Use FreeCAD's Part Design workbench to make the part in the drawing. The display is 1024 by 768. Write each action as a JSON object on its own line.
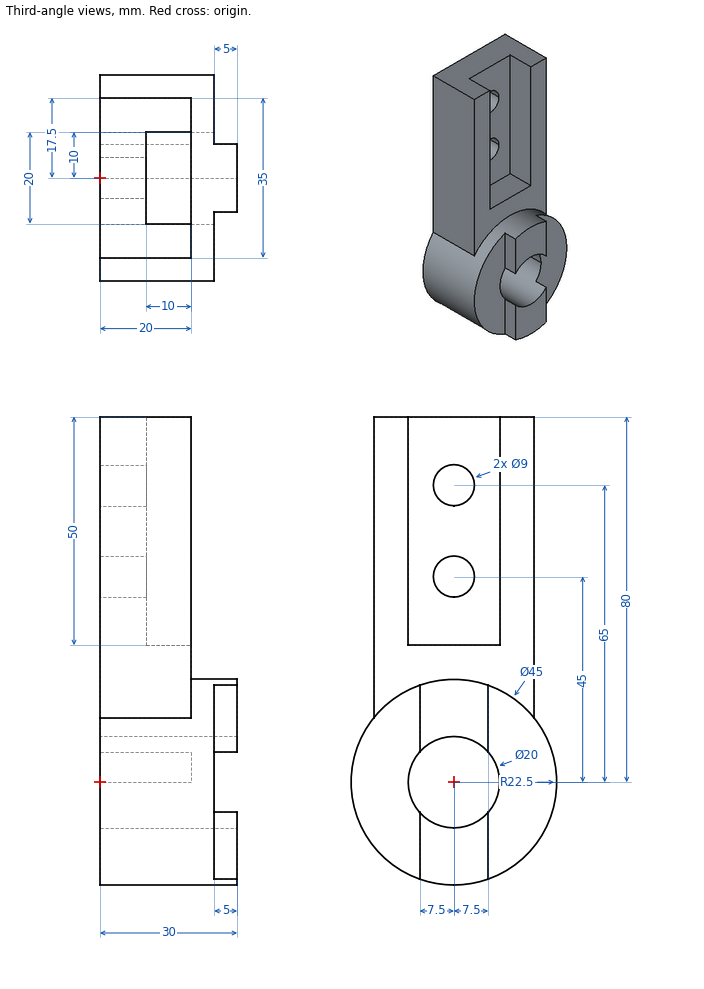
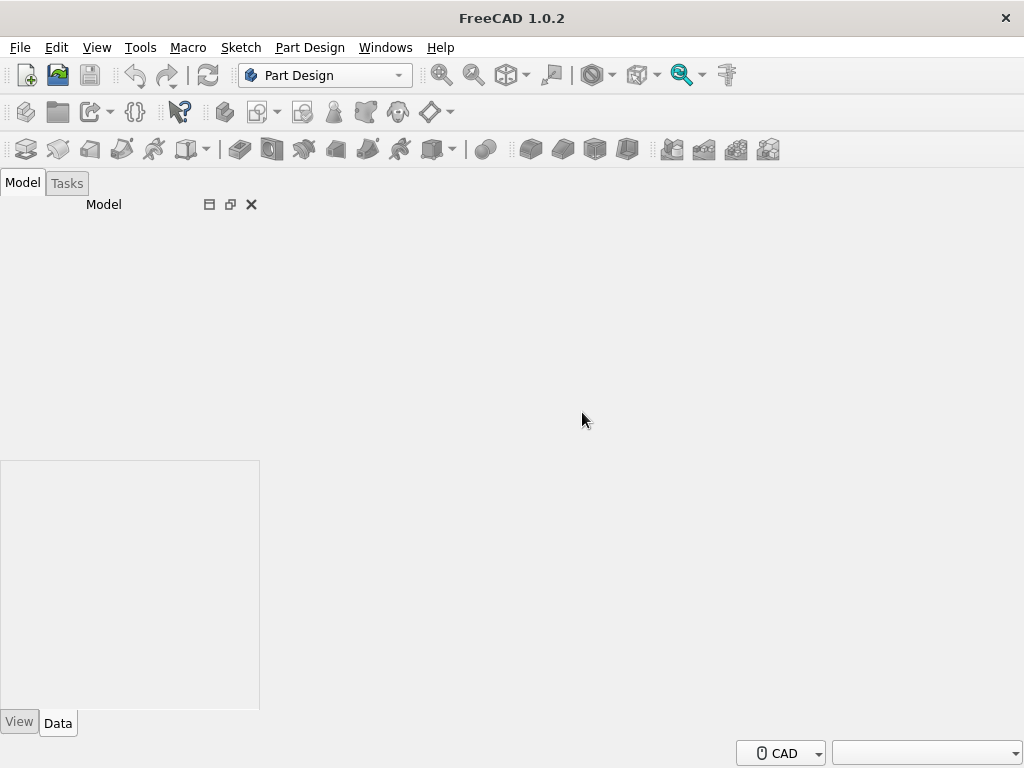
{"action": "left_click", "coordinate": [26, 76]}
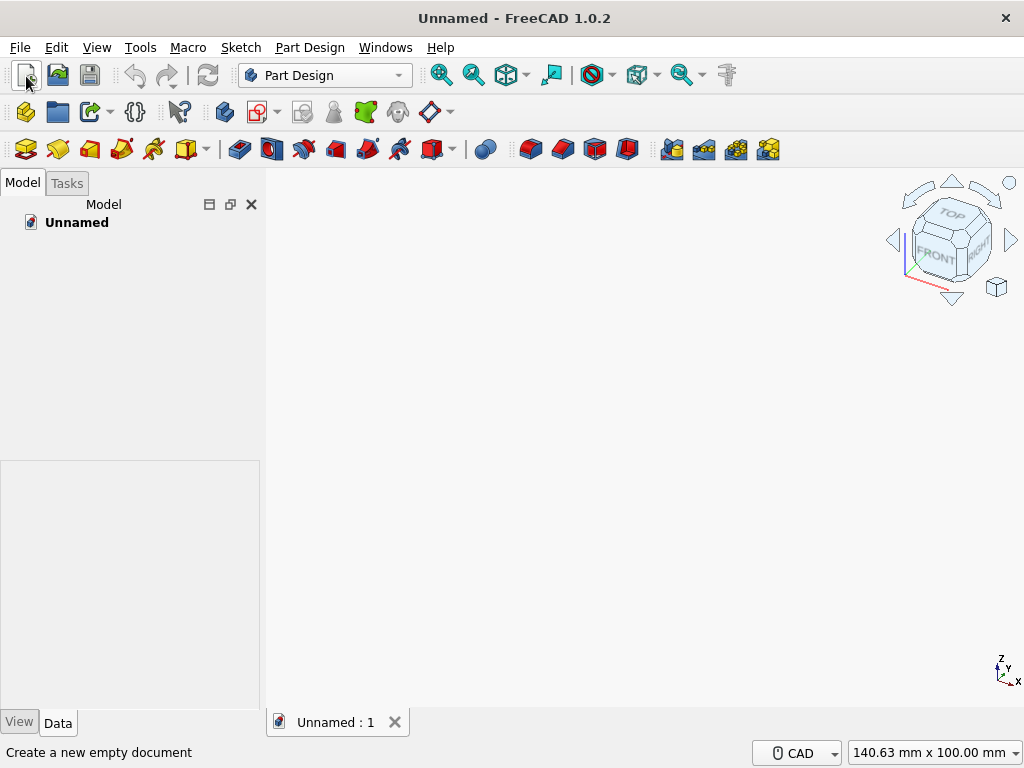
{"action": "left_click", "coordinate": [258, 112]}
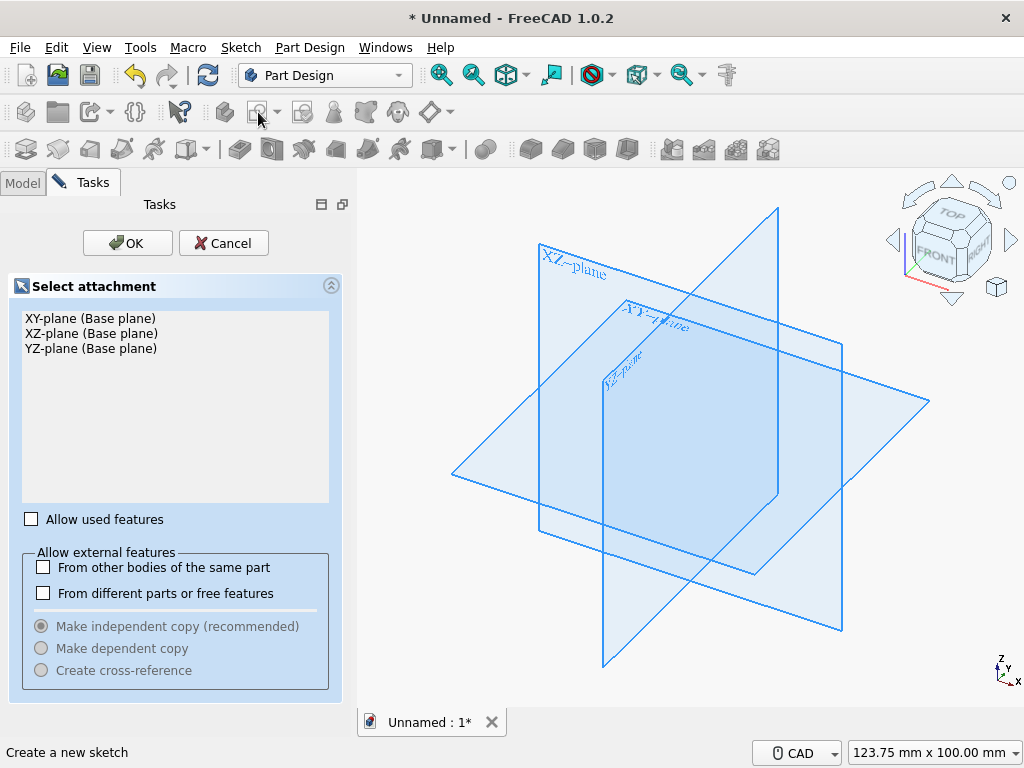
{"action": "left_click", "coordinate": [82, 348]}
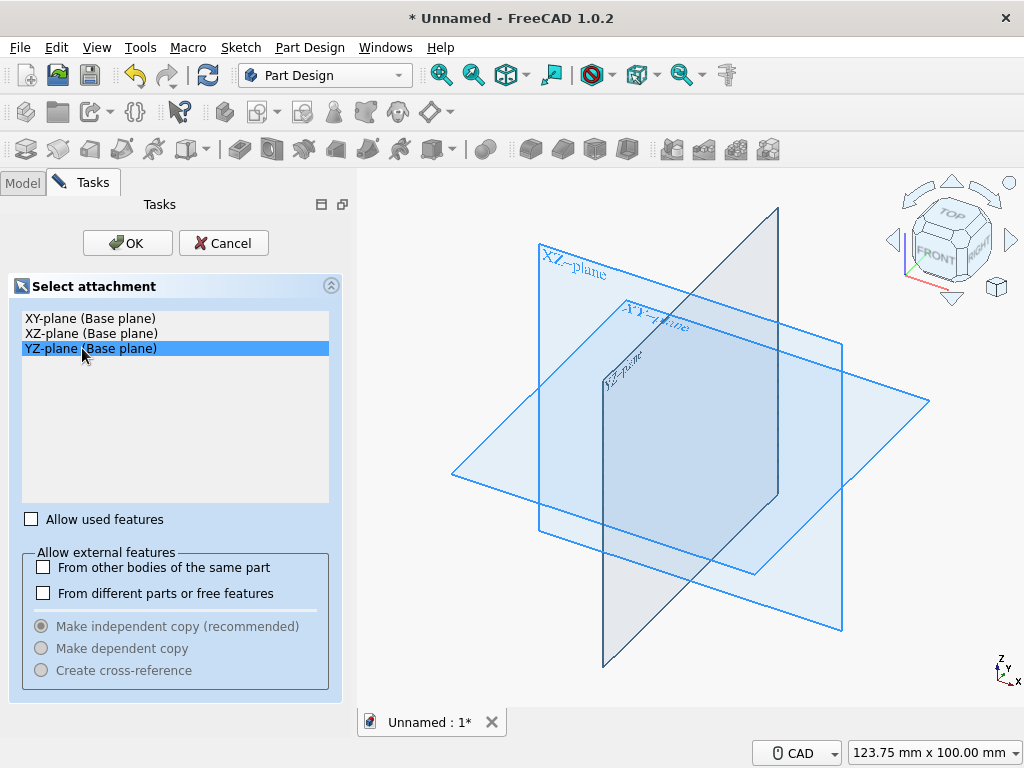
{"action": "left_click", "coordinate": [128, 243]}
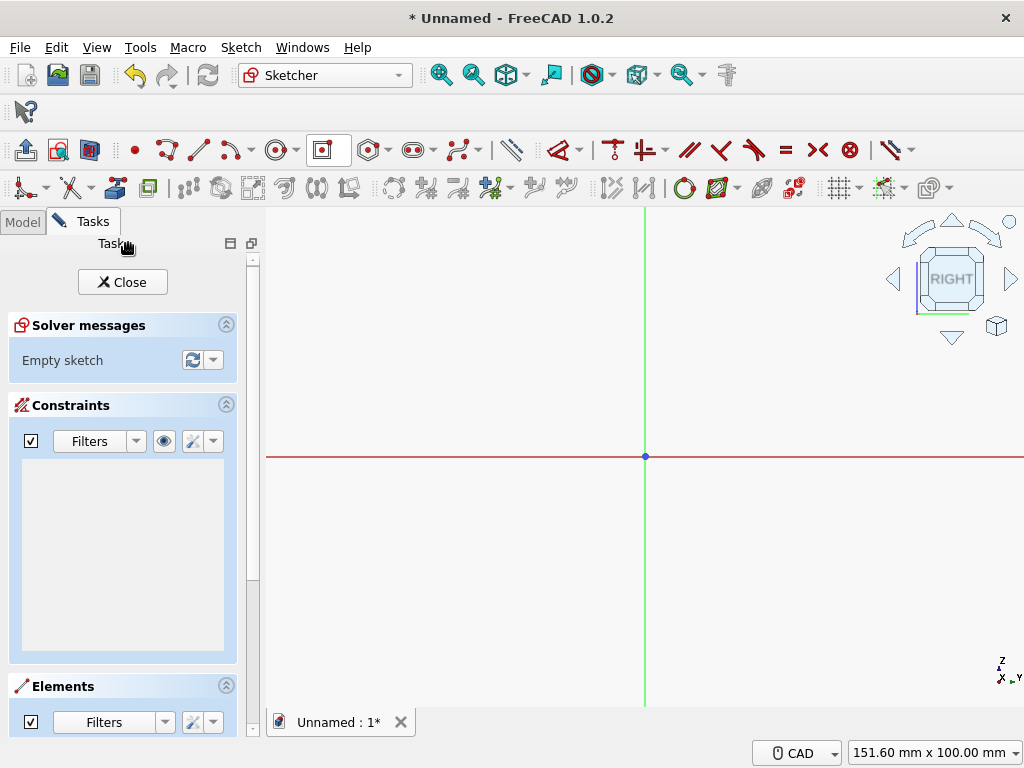
{"action": "scroll", "coordinate": [784, 457], "scroll_direction": "up", "scroll_amount": 2}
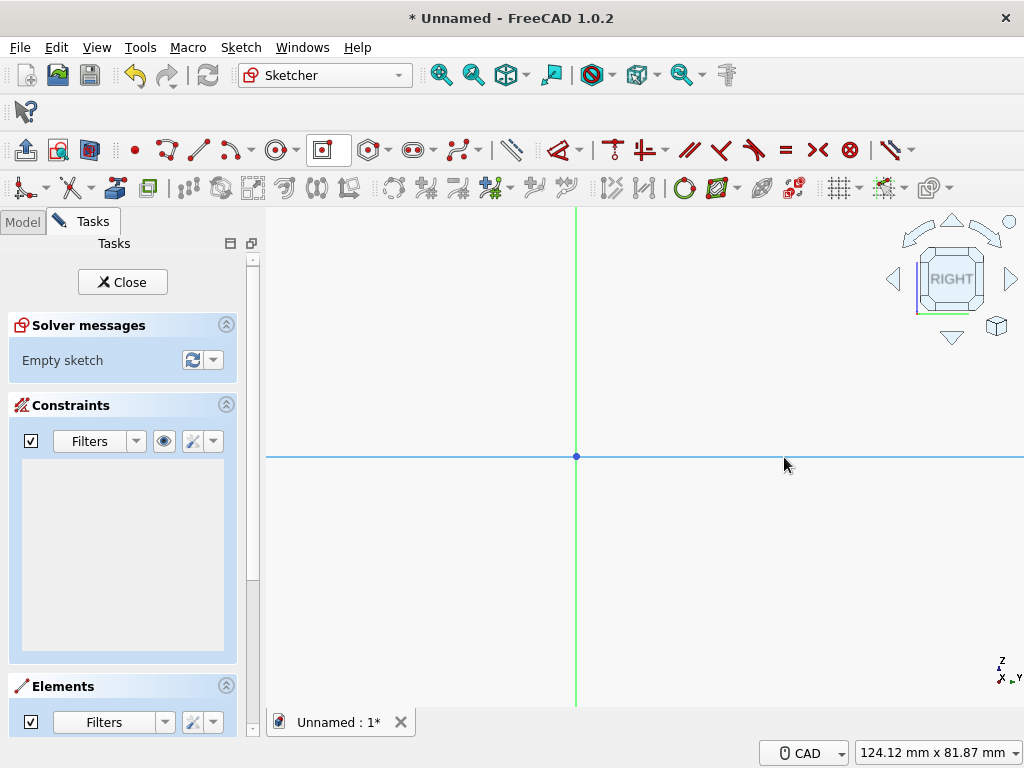
{"action": "left_click", "coordinate": [276, 150]}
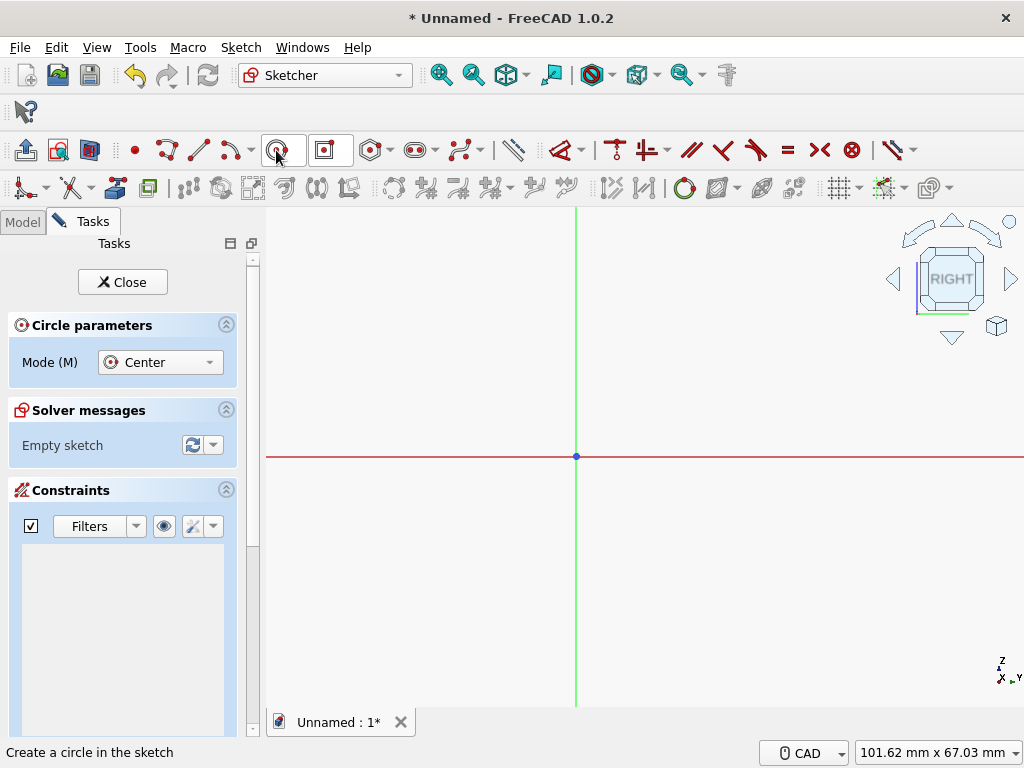
{"action": "left_click", "coordinate": [576, 457]}
{"action": "mouse_move", "coordinate": [695, 338]}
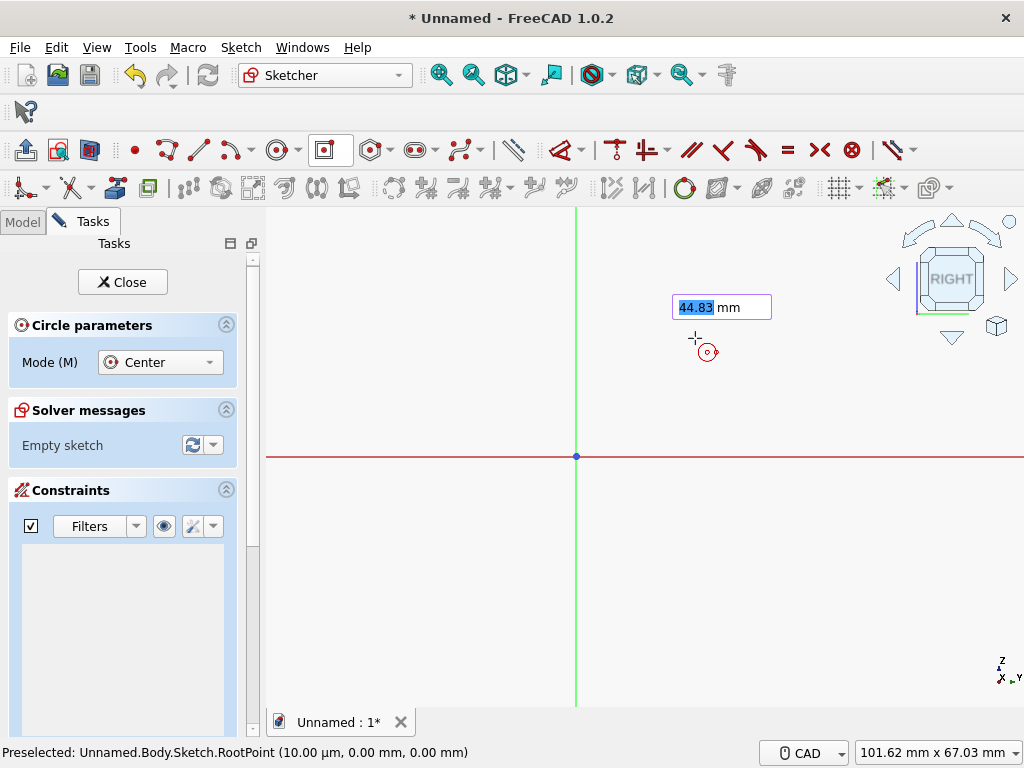
{"action": "type", "text": "45"}
{"action": "key", "text": "Return"}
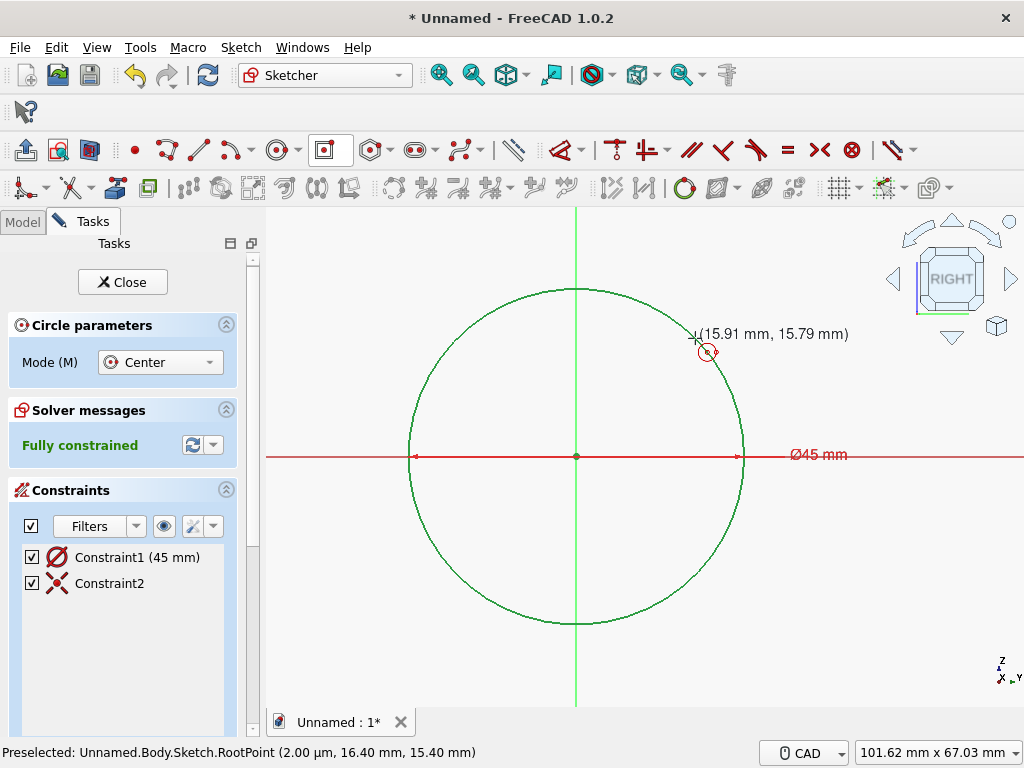
{"action": "left_click", "coordinate": [576, 457]}
{"action": "mouse_move", "coordinate": [629, 404]}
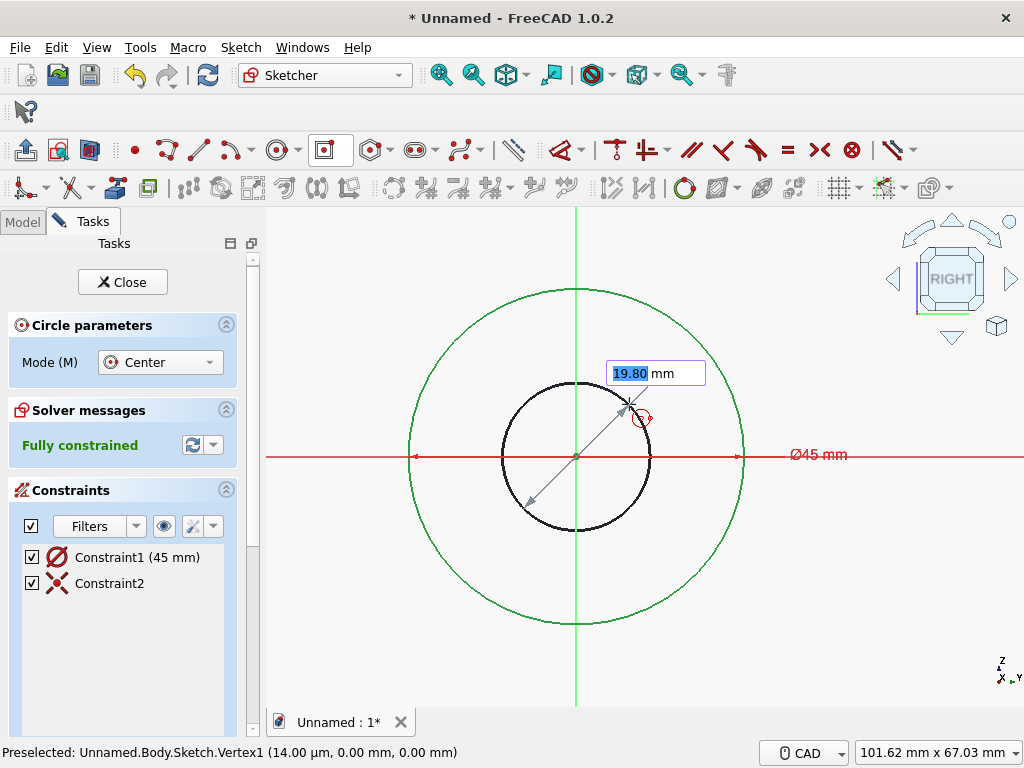
{"action": "type", "text": "20"}
{"action": "key", "text": "Return"}
{"action": "key", "text": "Escape"}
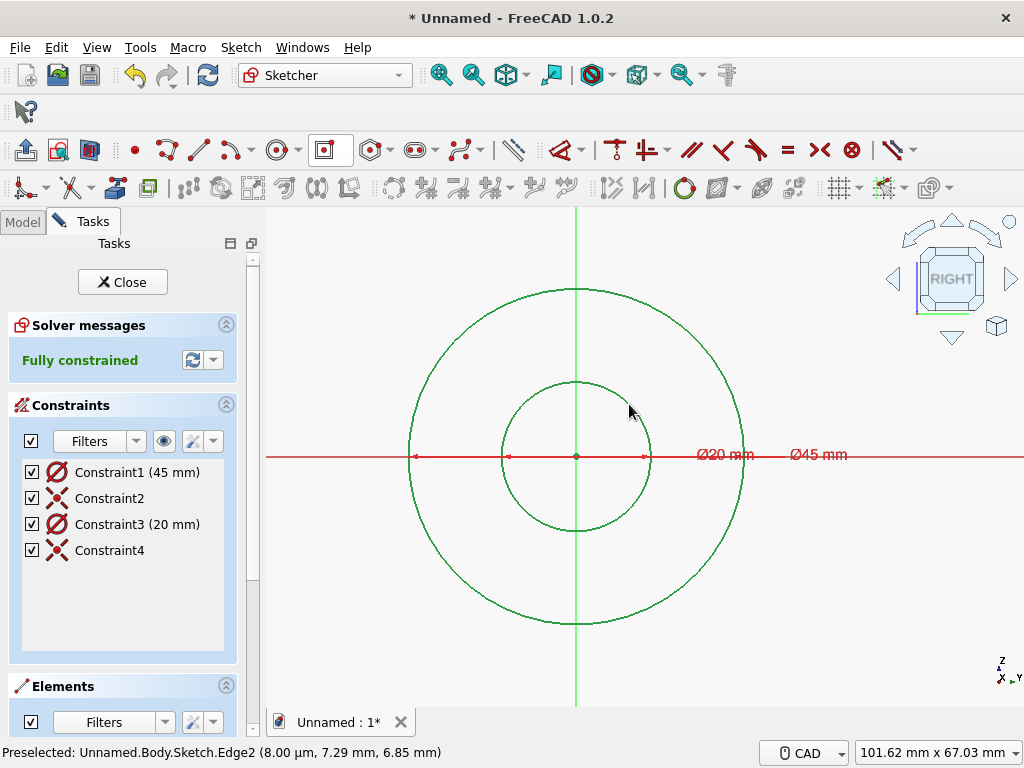
{"action": "left_click", "coordinate": [123, 282]}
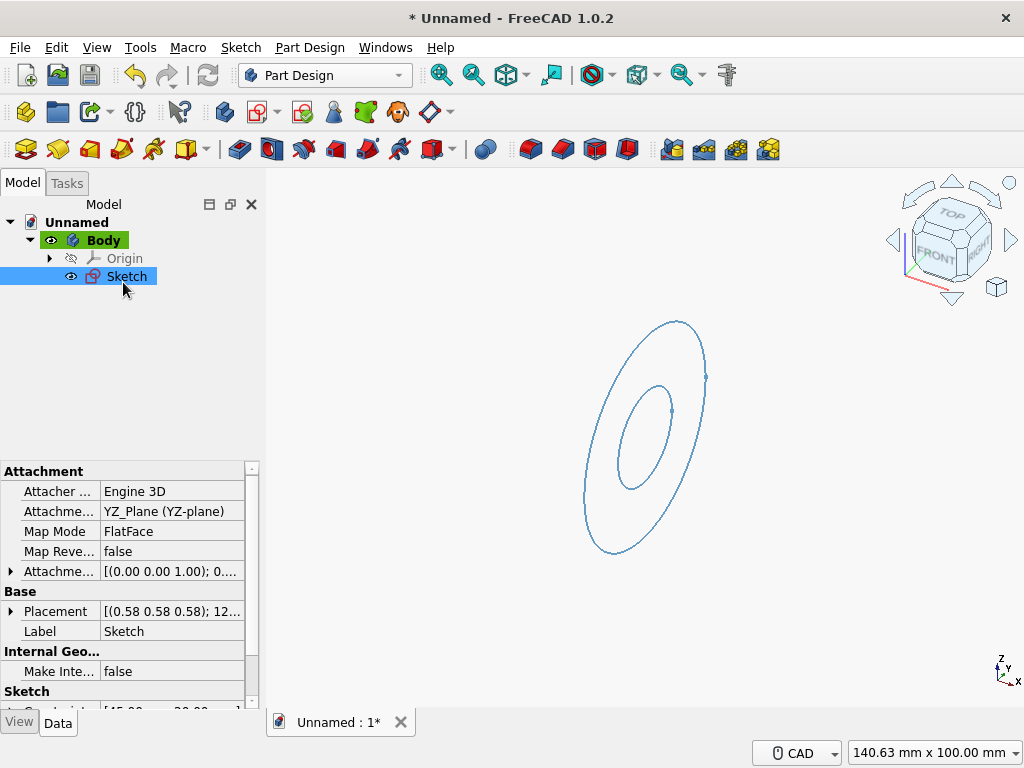
{"action": "left_click", "coordinate": [26, 150]}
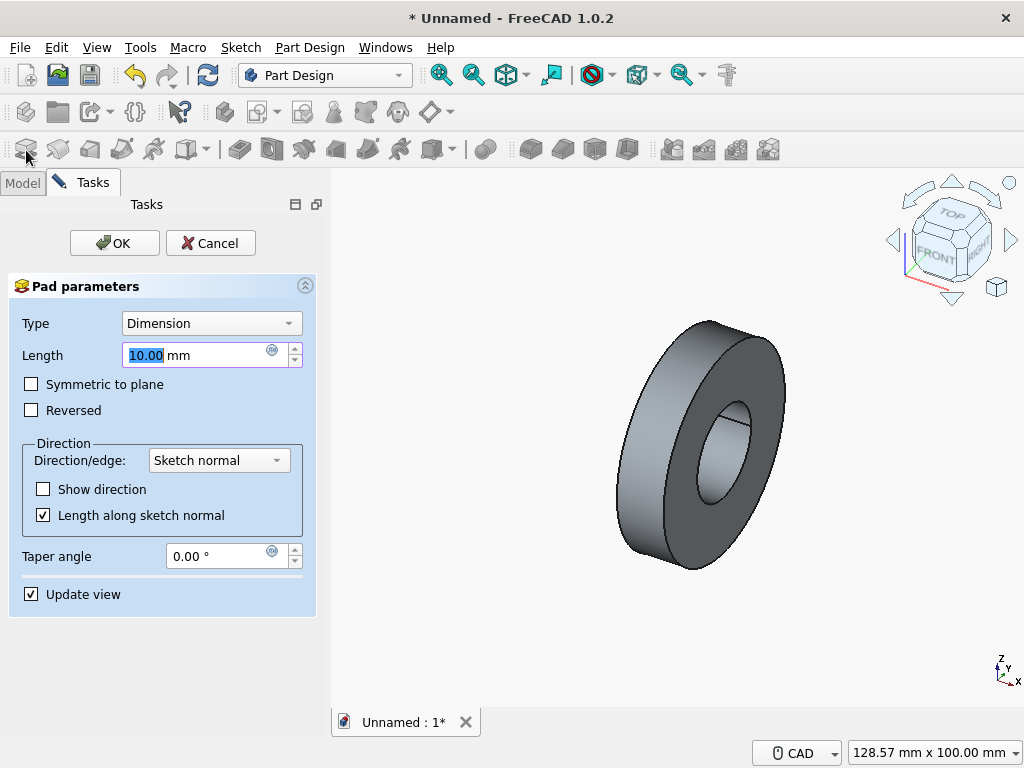
{"action": "type", "text": "30"}
{"action": "key", "text": "Tab"}